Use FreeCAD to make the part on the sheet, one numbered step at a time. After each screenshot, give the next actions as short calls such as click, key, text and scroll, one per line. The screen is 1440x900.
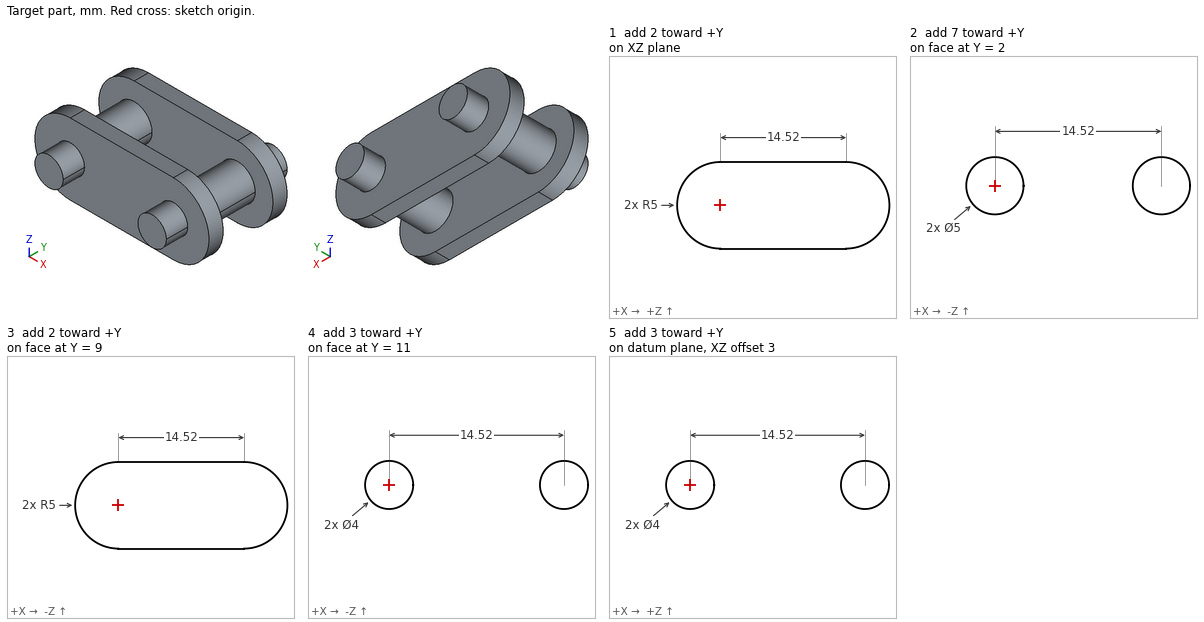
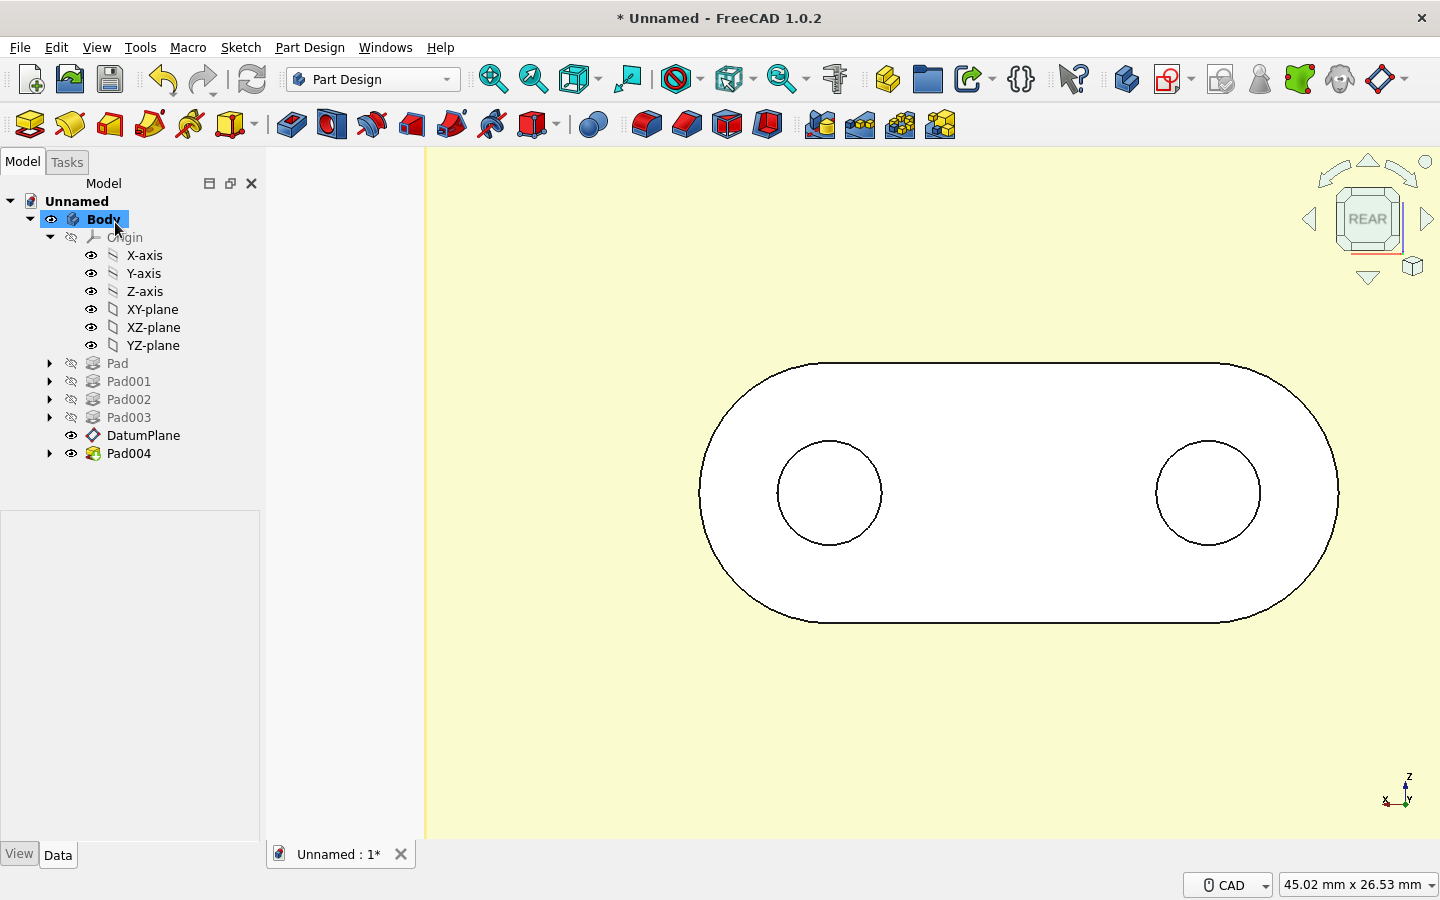
click(116, 435)
key(space)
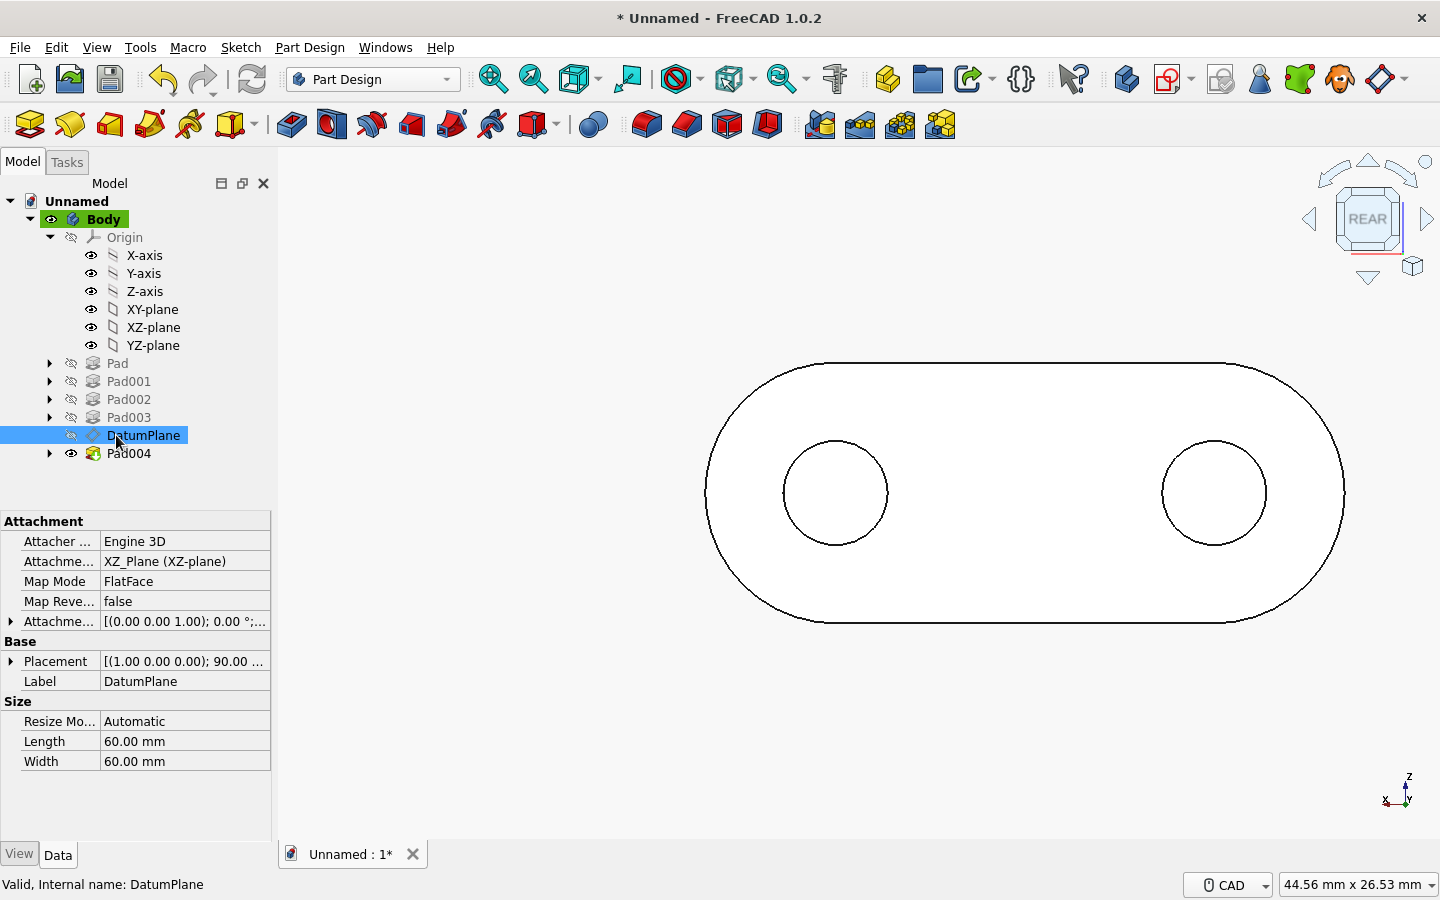
key(0)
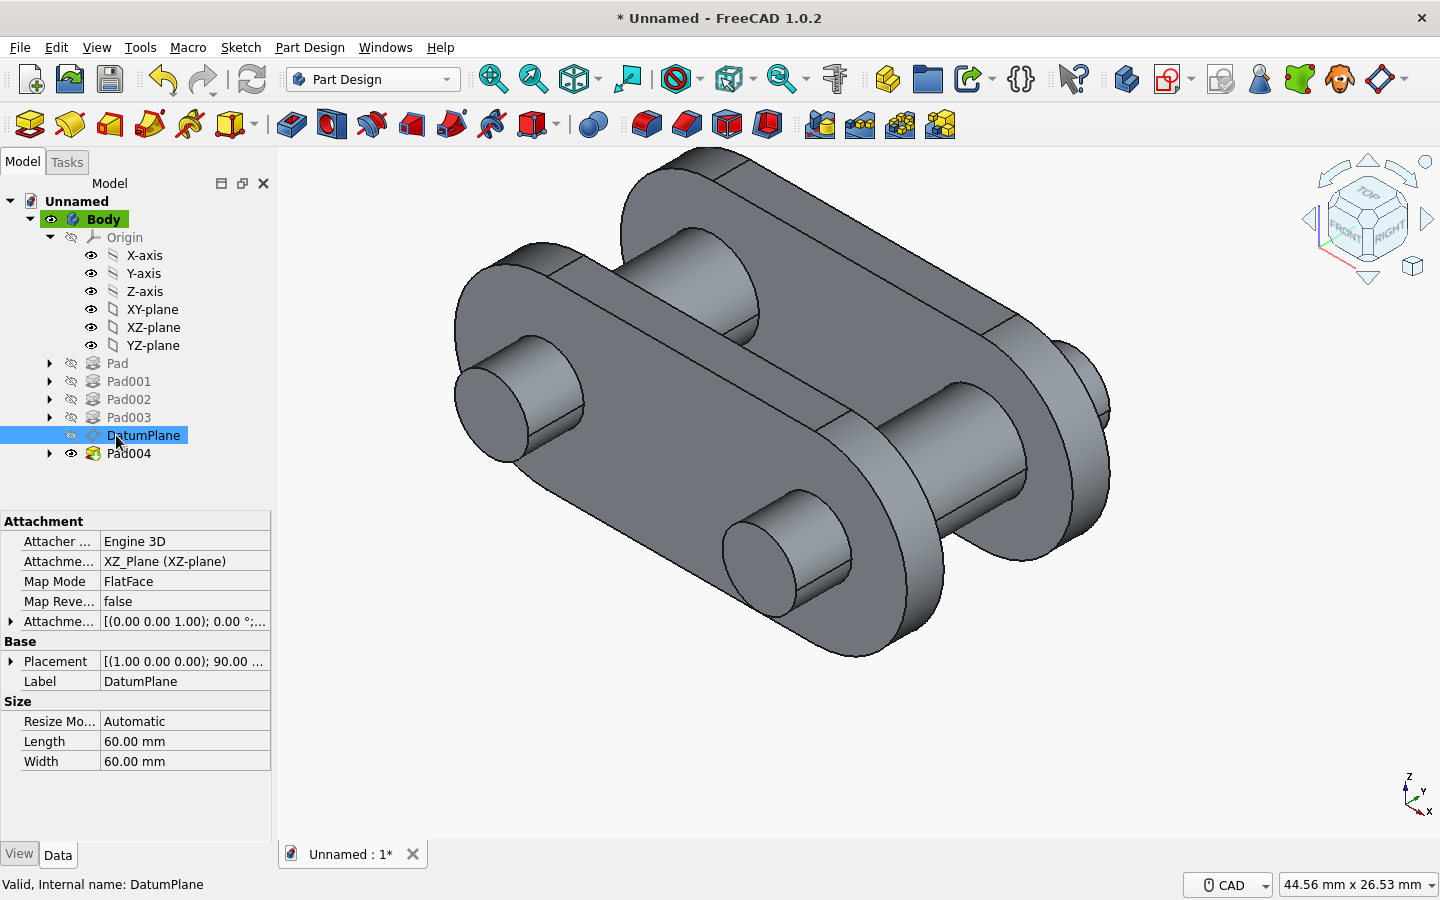
key(v)
key(f)